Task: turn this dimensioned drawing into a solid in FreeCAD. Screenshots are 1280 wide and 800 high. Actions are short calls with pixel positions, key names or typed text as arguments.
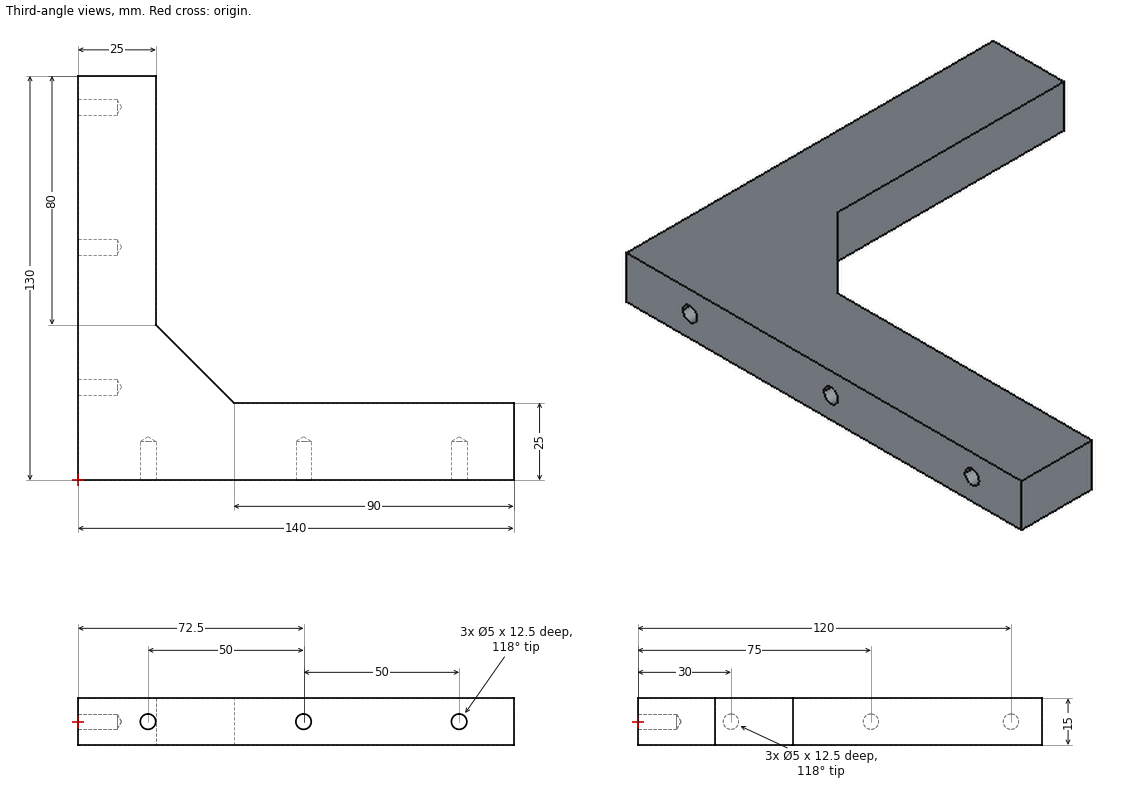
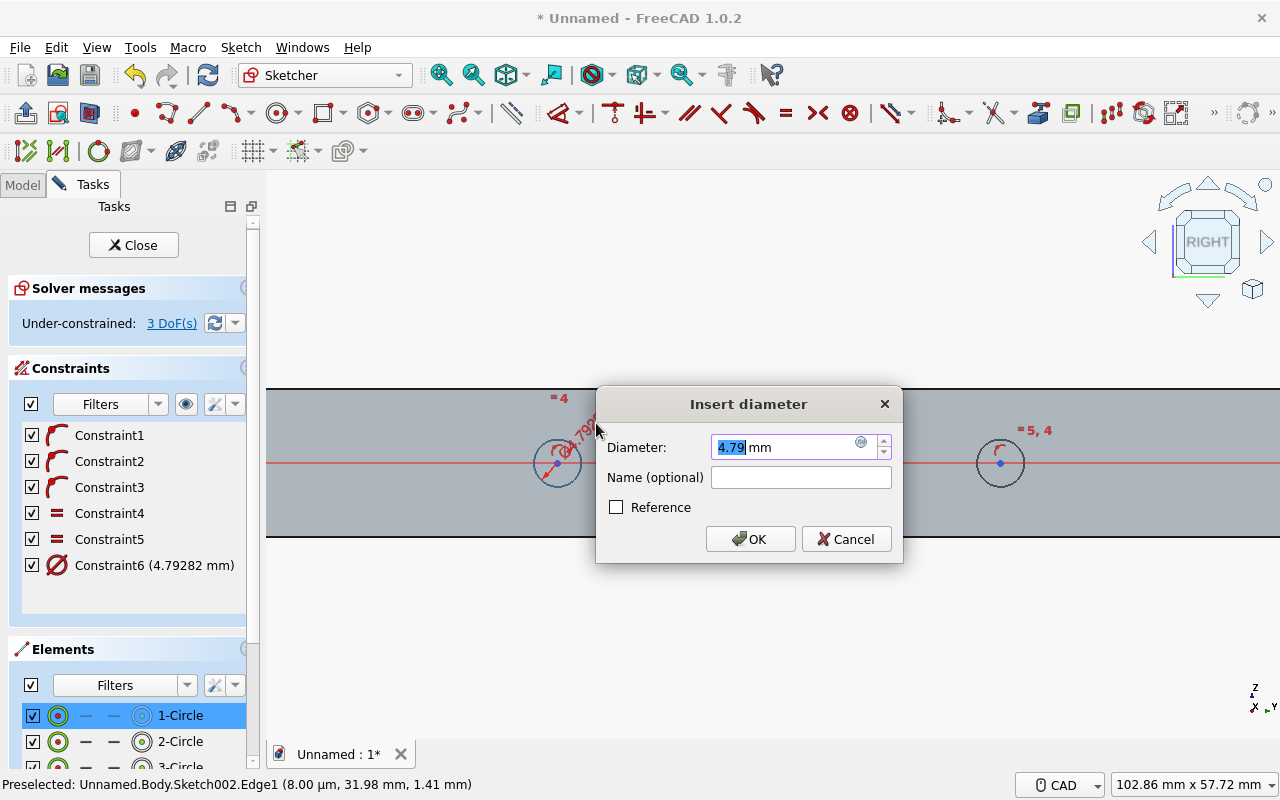
text(5)
key(Return)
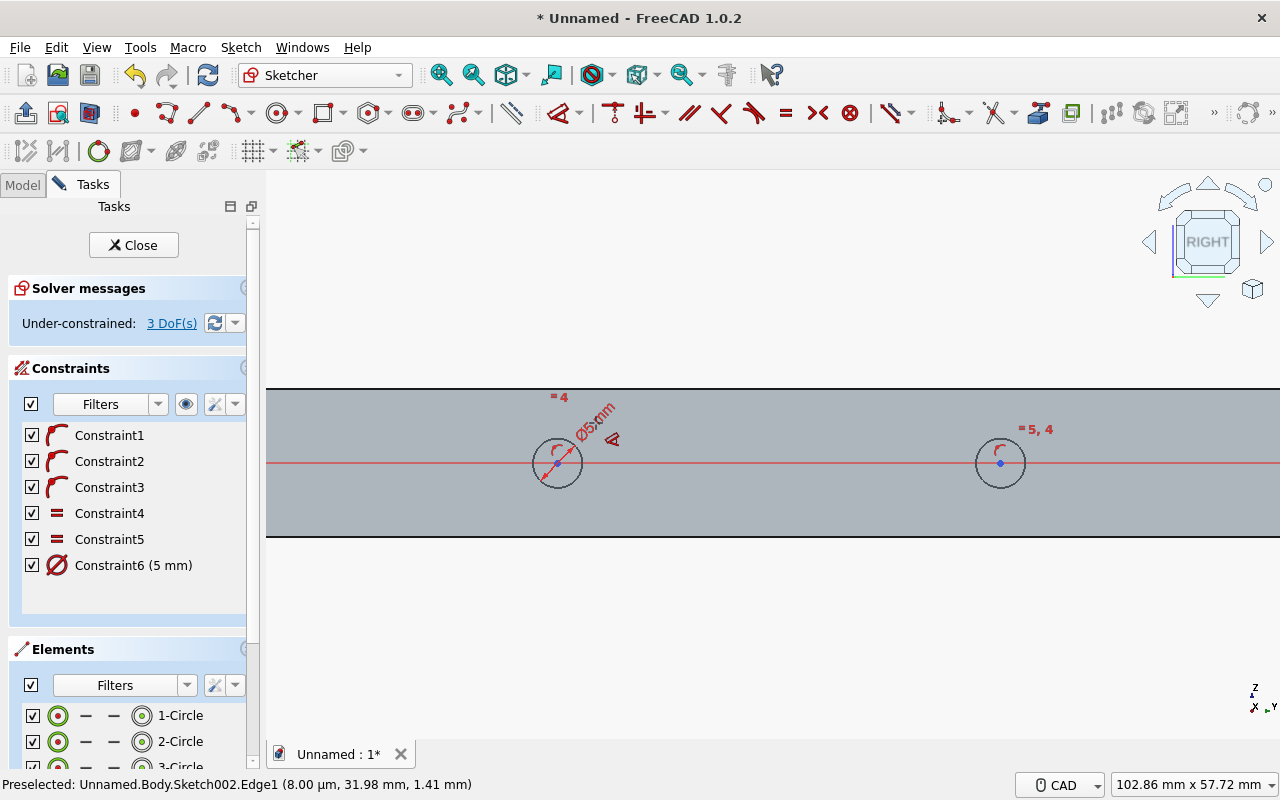
click(558, 463)
click(426, 497)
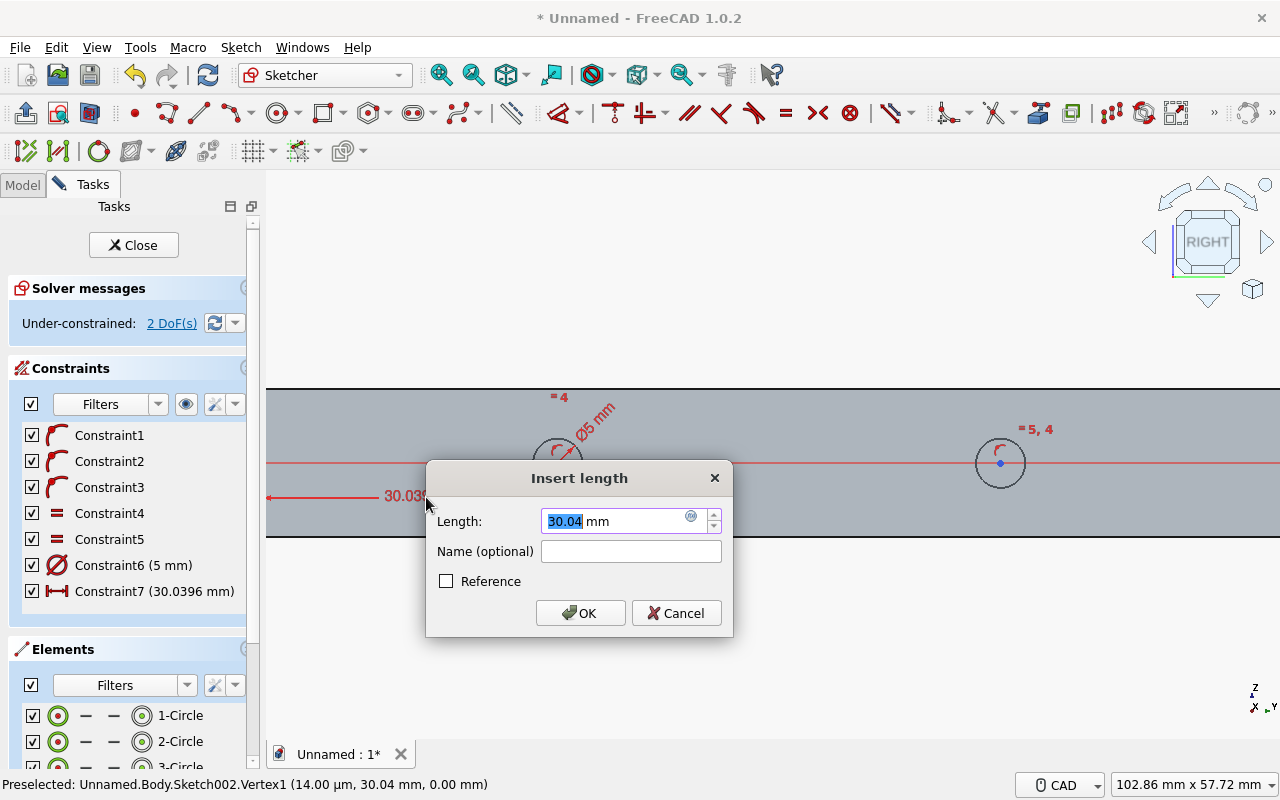
text(30)
key(Return)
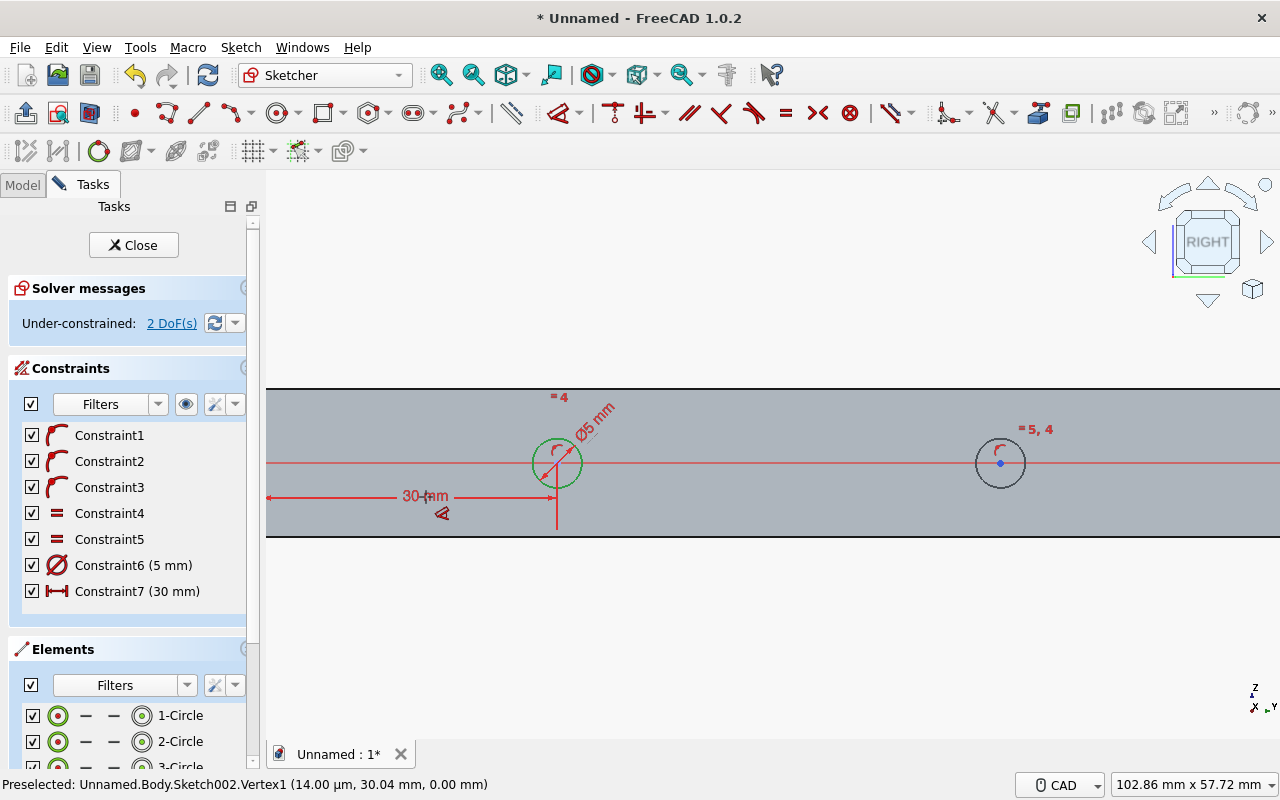
click(1001, 463)
click(647, 497)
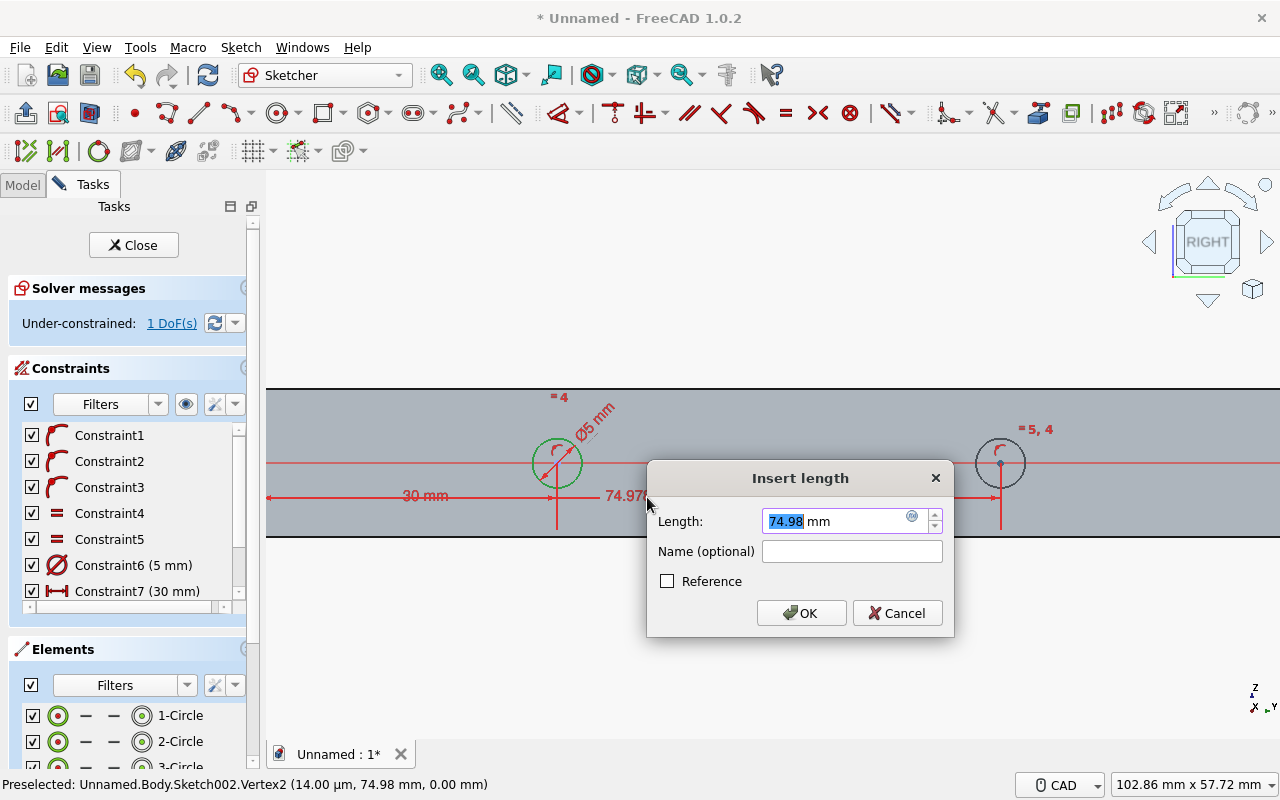
text(75)
key(Return)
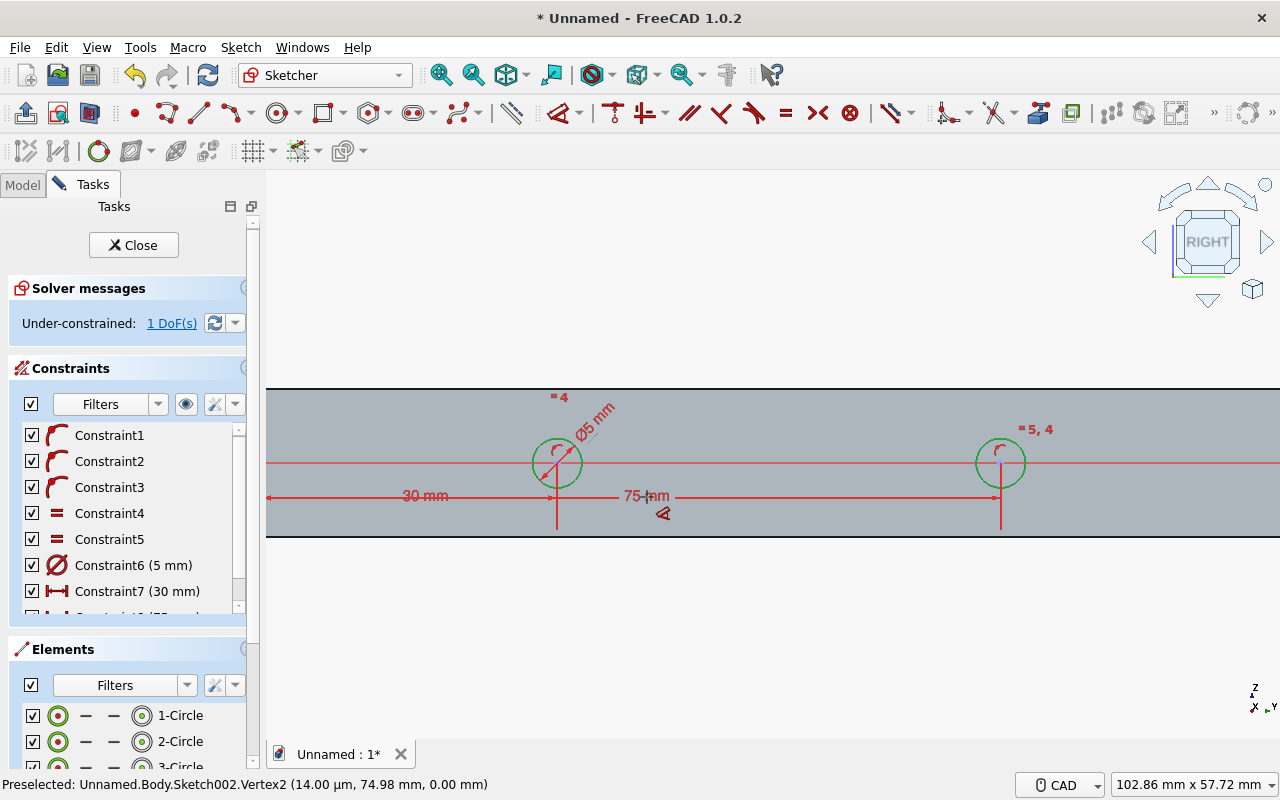
scroll(573, 447, down, 4)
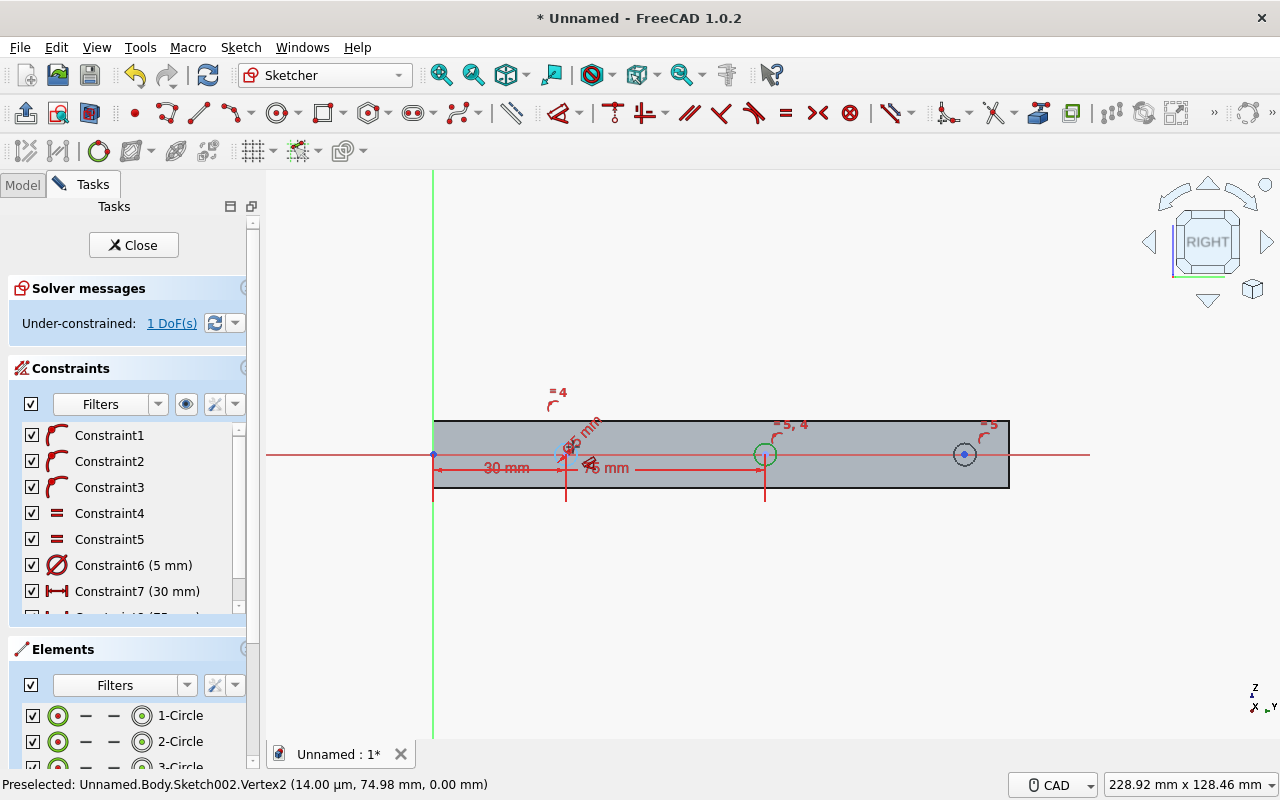
click(965, 455)
click(699, 489)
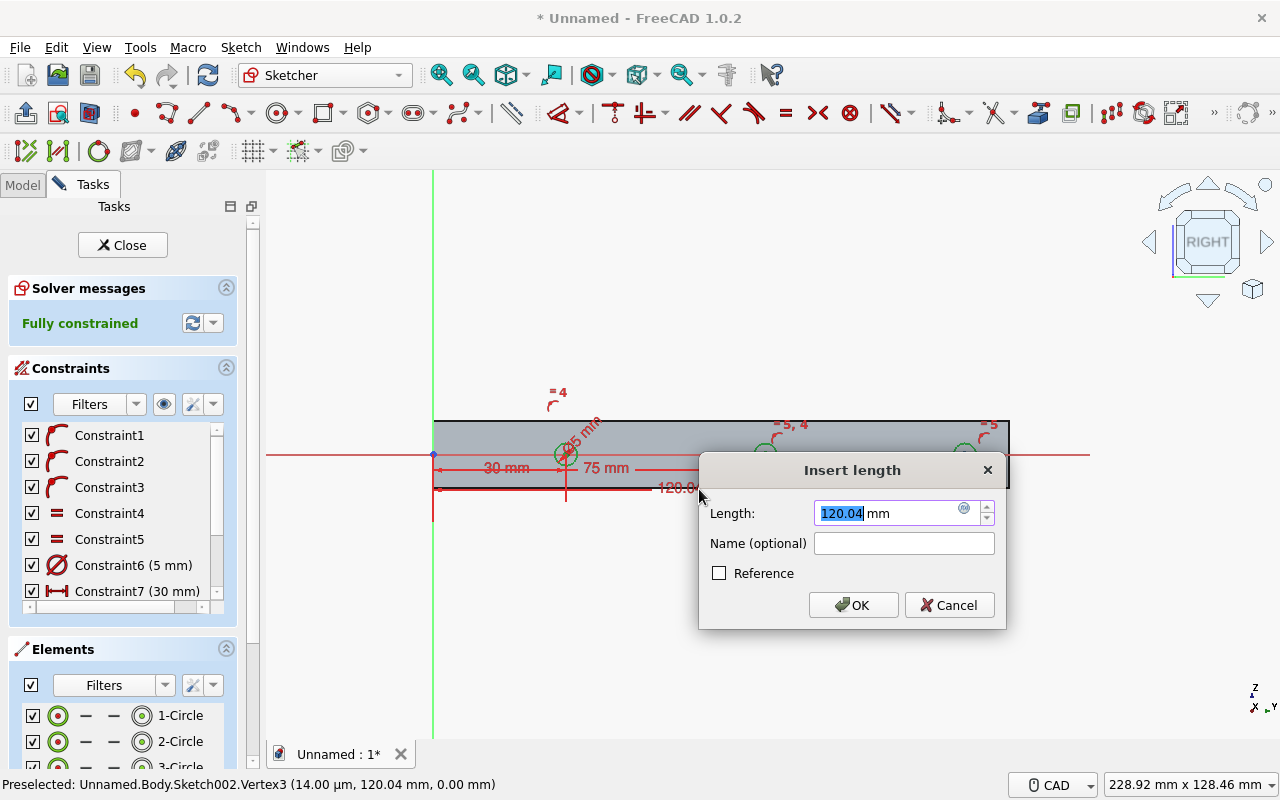
text(120)
key(Return)
key(Escape)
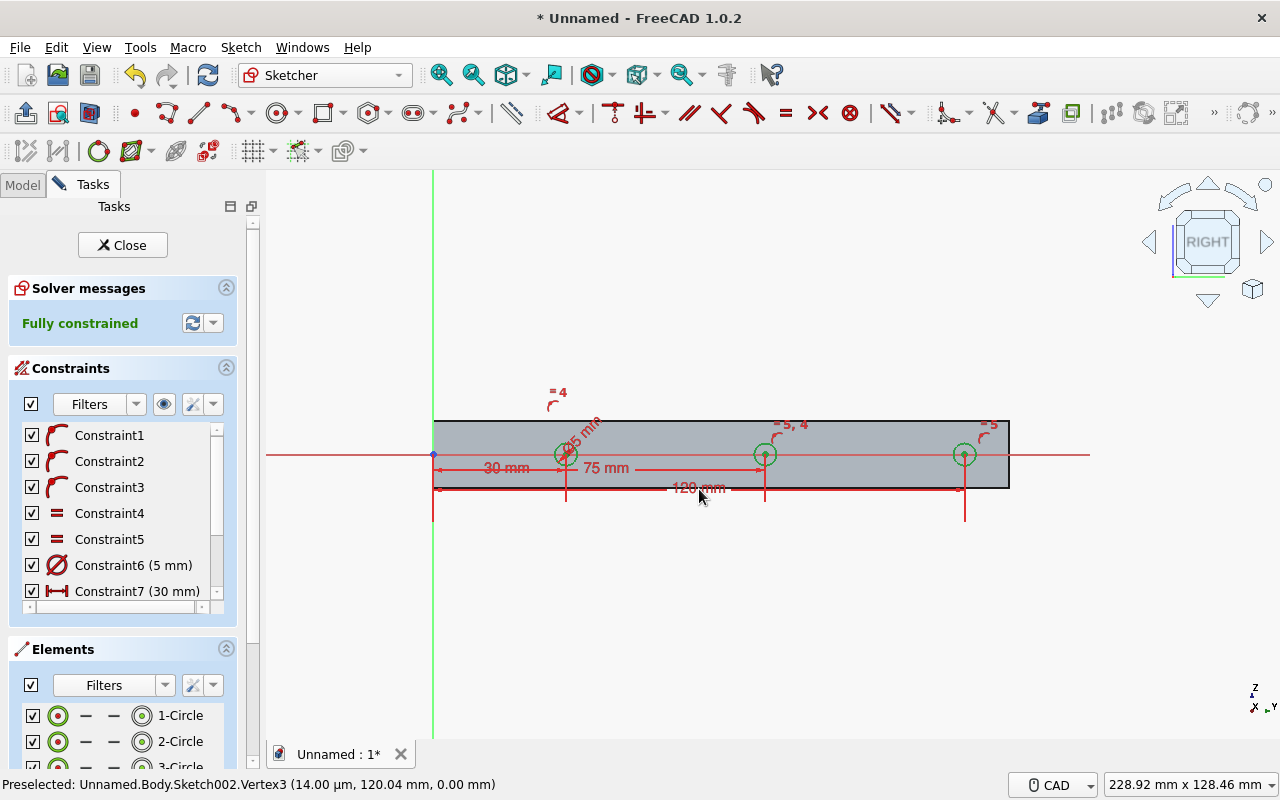
click(123, 245)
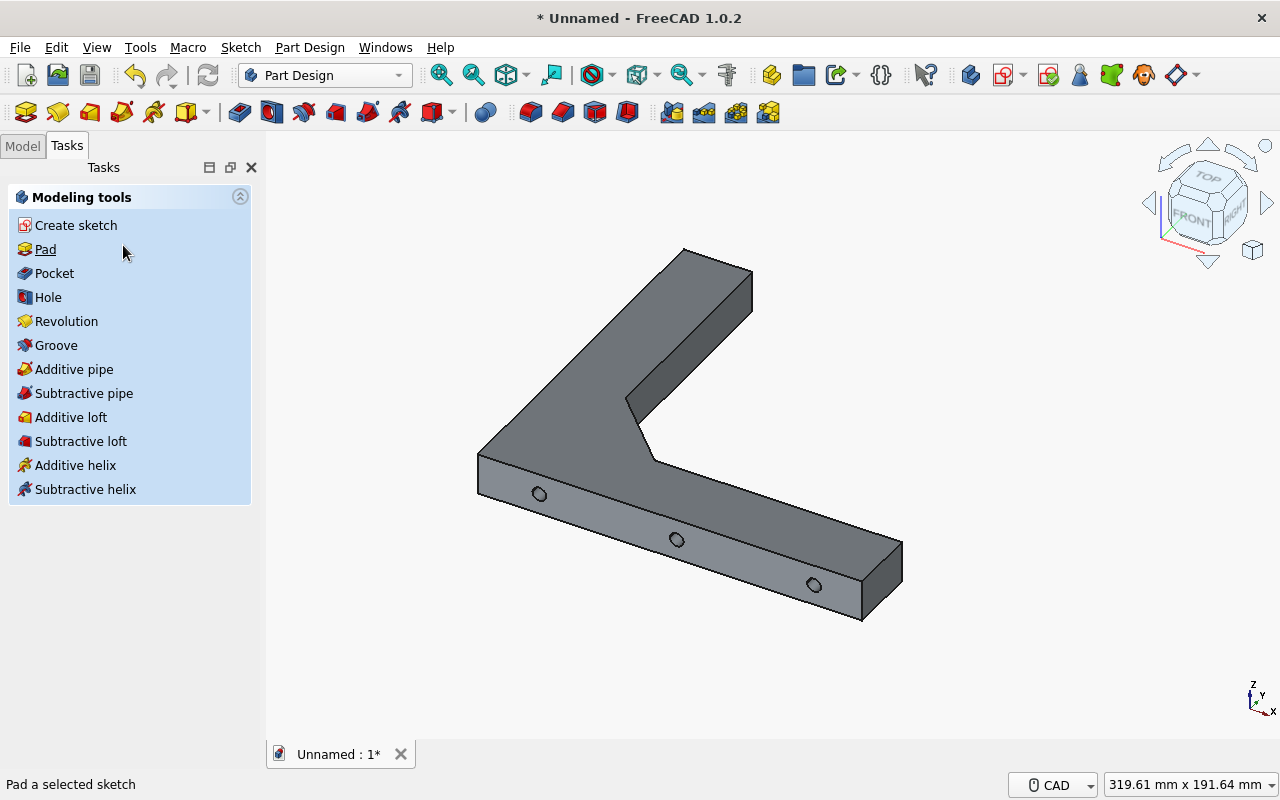
click(272, 112)